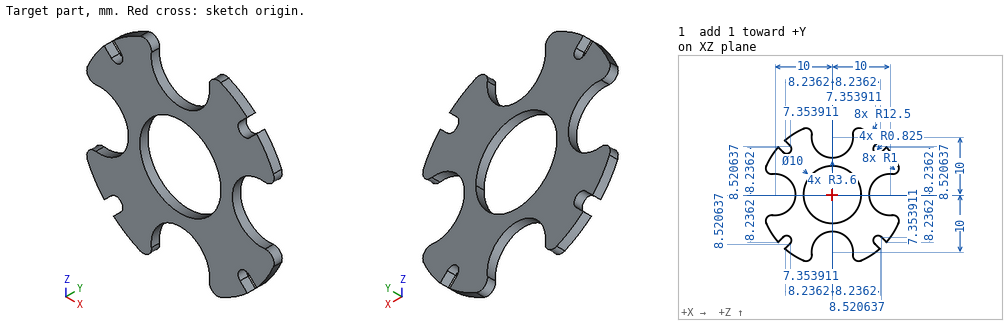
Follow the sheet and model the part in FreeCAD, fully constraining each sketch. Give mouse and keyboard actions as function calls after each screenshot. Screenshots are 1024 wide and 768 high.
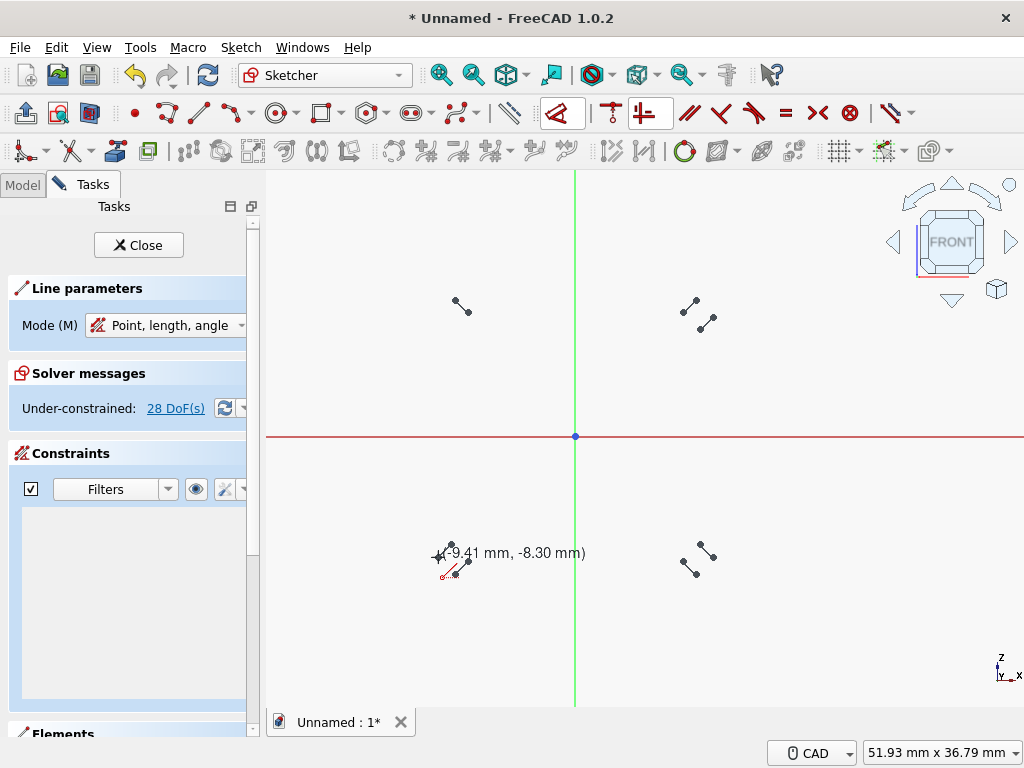
click(438, 317)
click(451, 329)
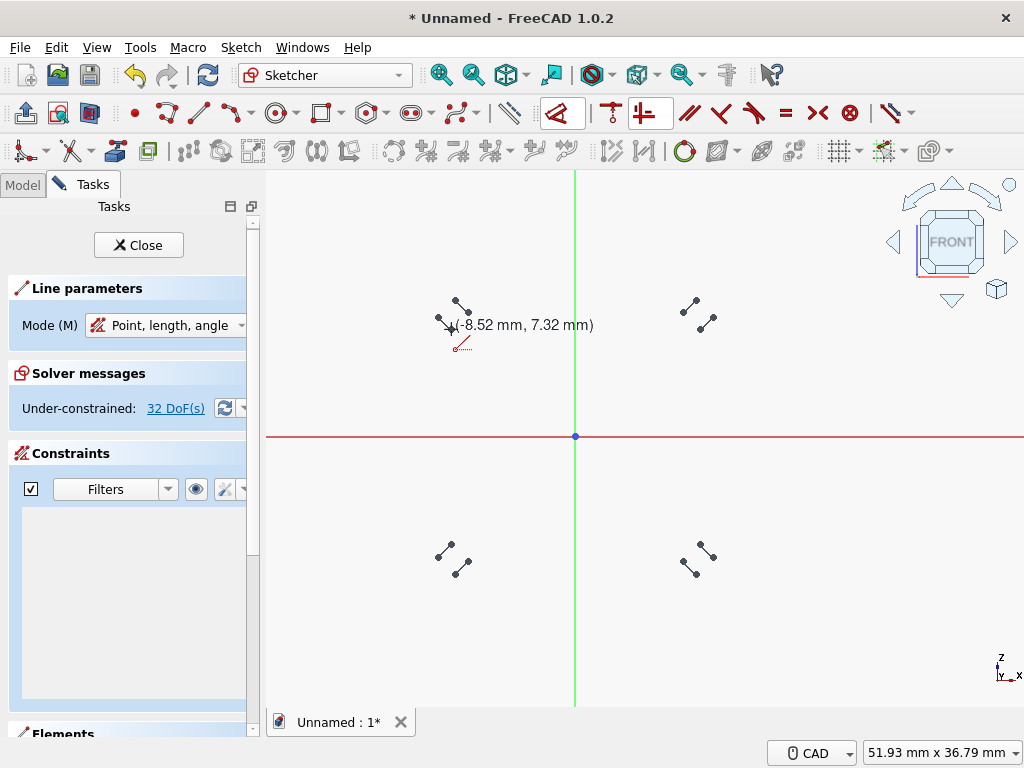
click(232, 114)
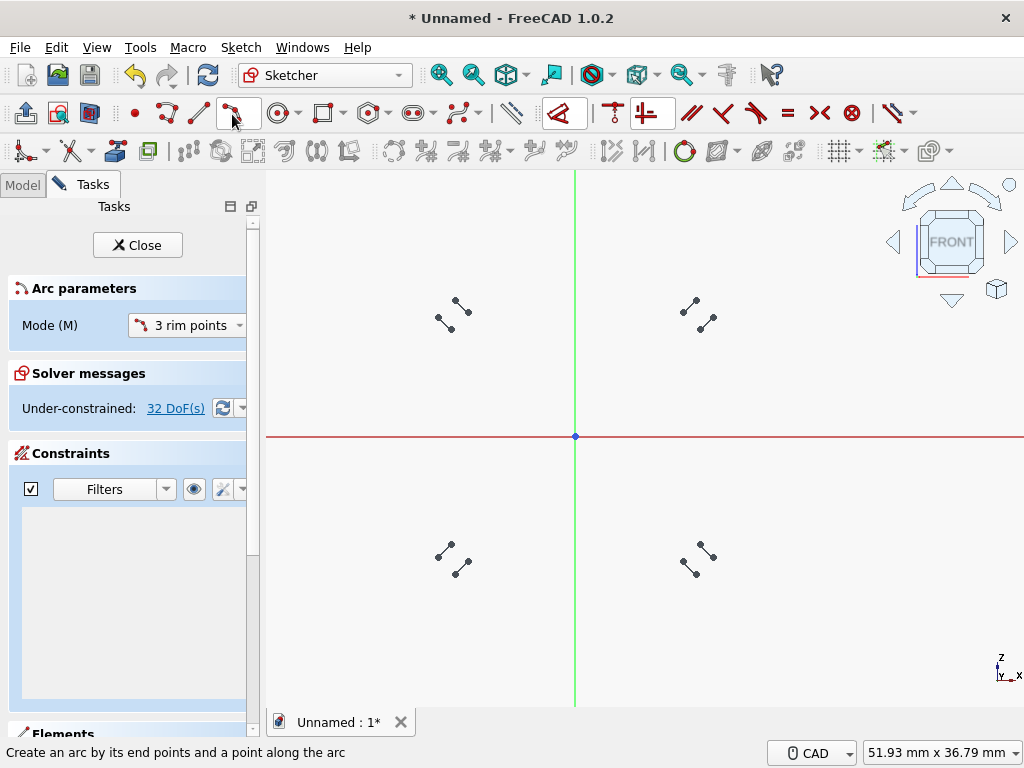
scroll(455, 300, up, 3)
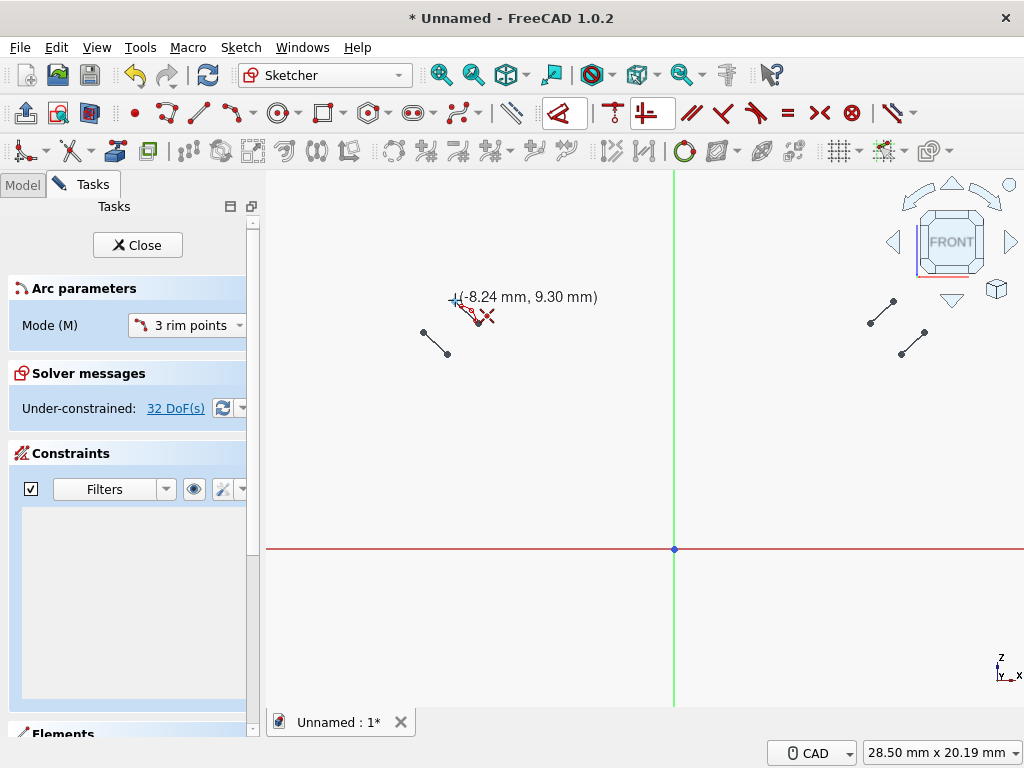
click(455, 302)
click(542, 244)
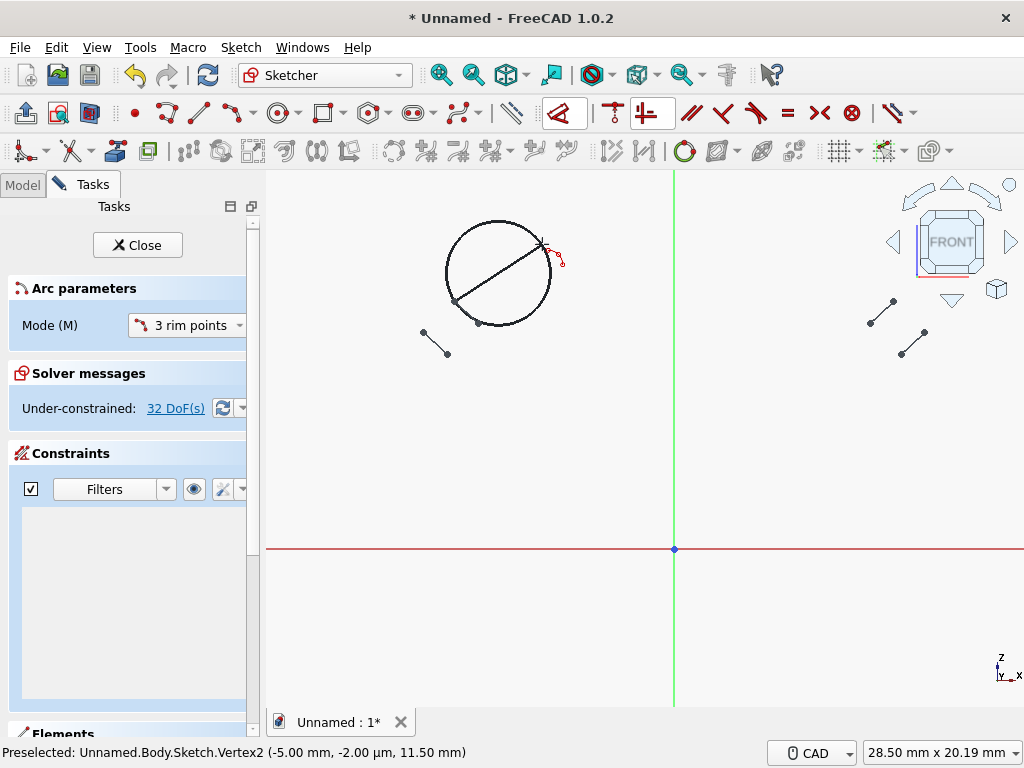
scroll(496, 268, up, 7)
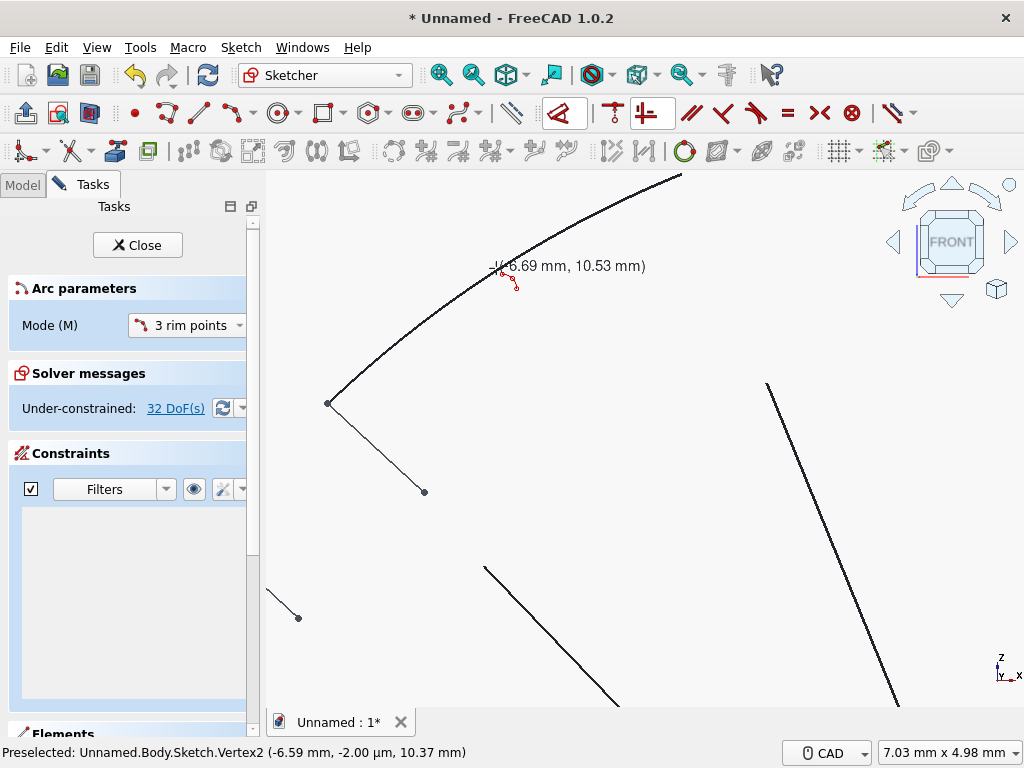
click(496, 268)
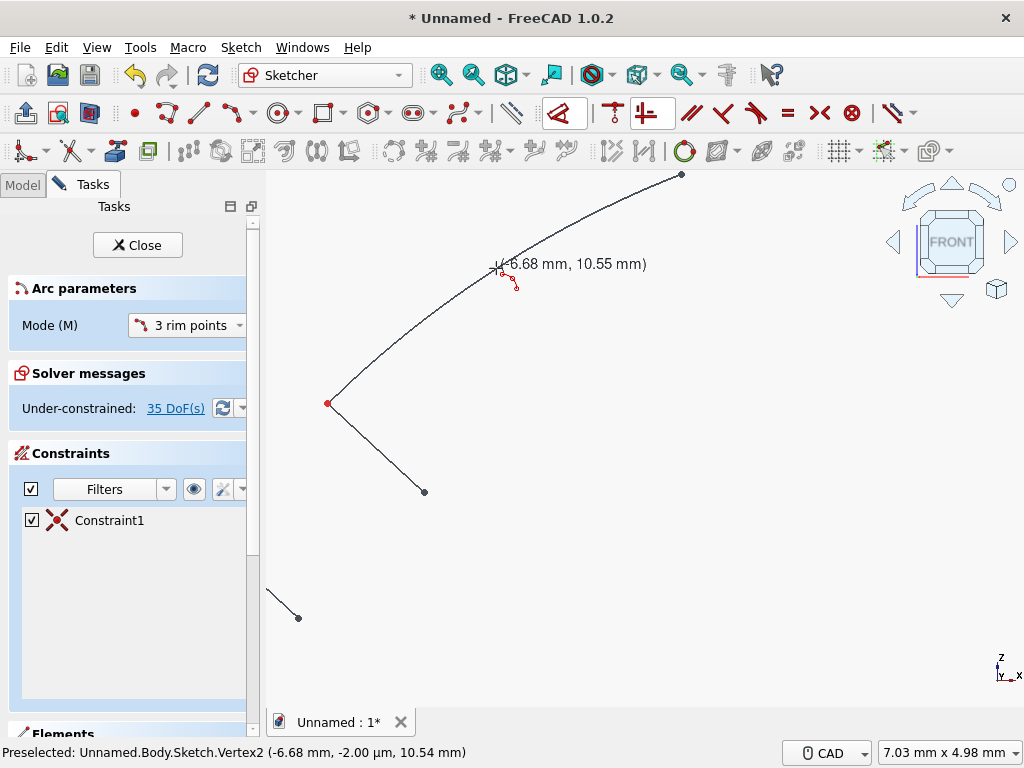
scroll(476, 287, down, 10)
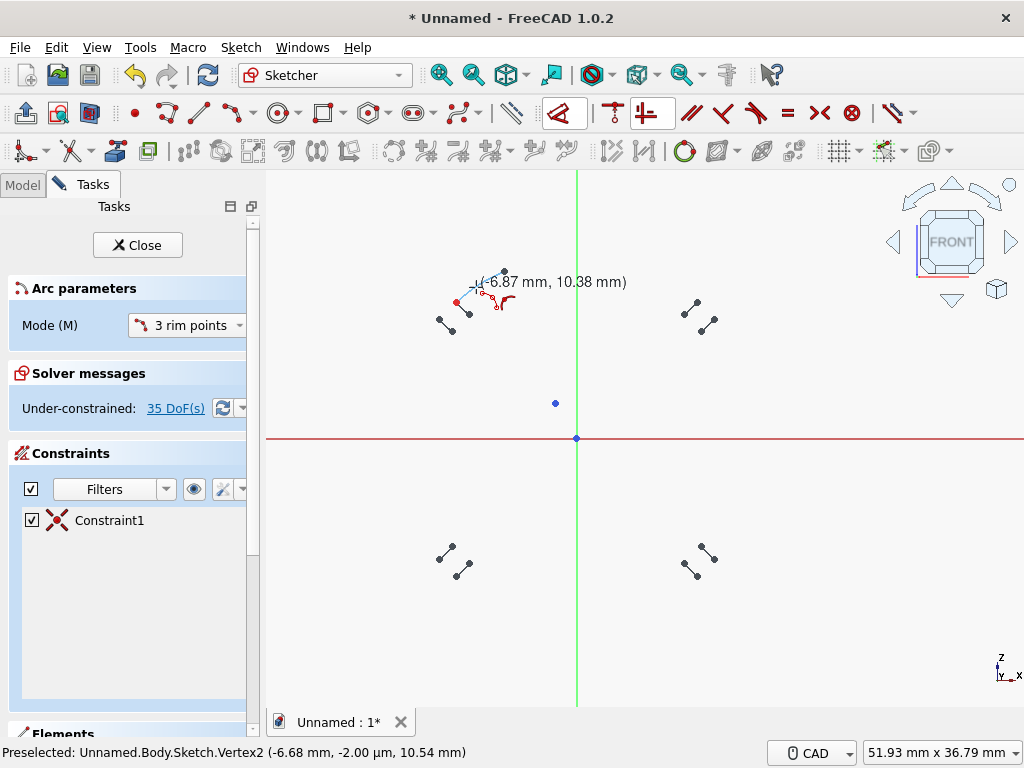
click(504, 272)
click(524, 286)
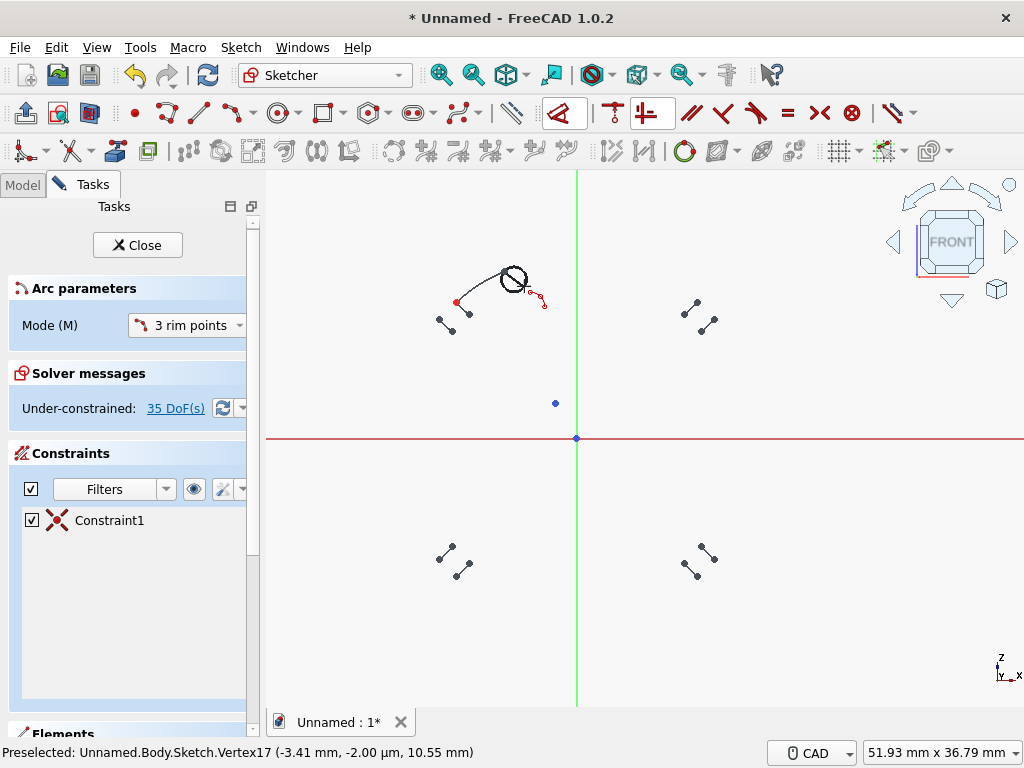
scroll(519, 273, up, 4)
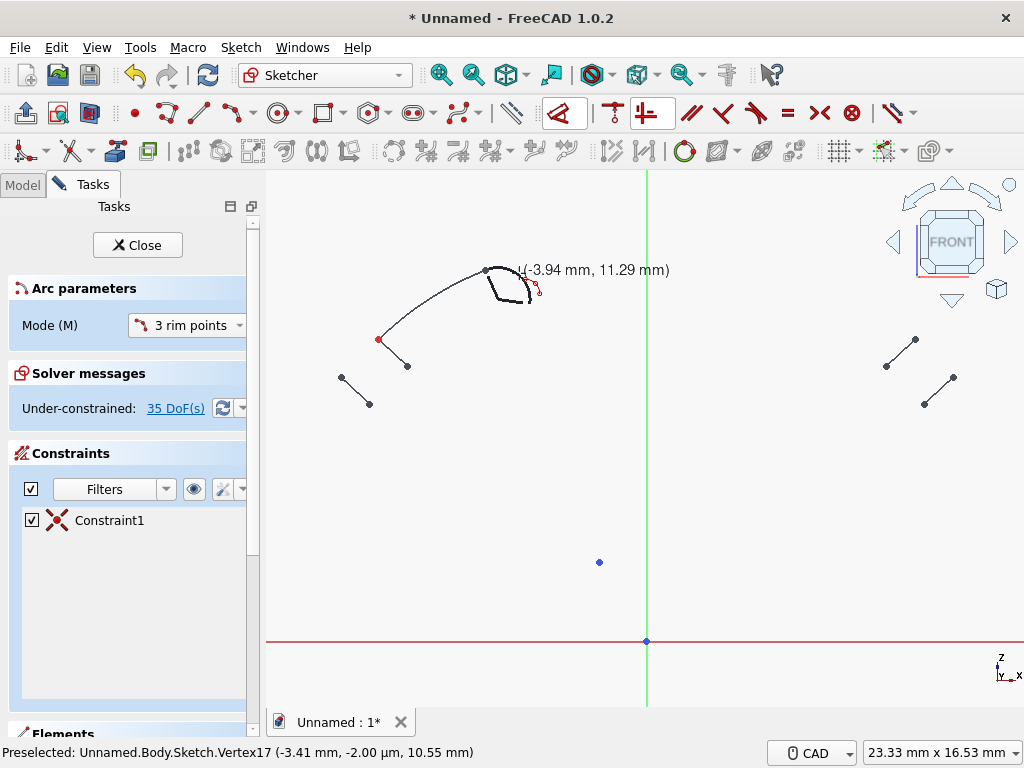
click(518, 273)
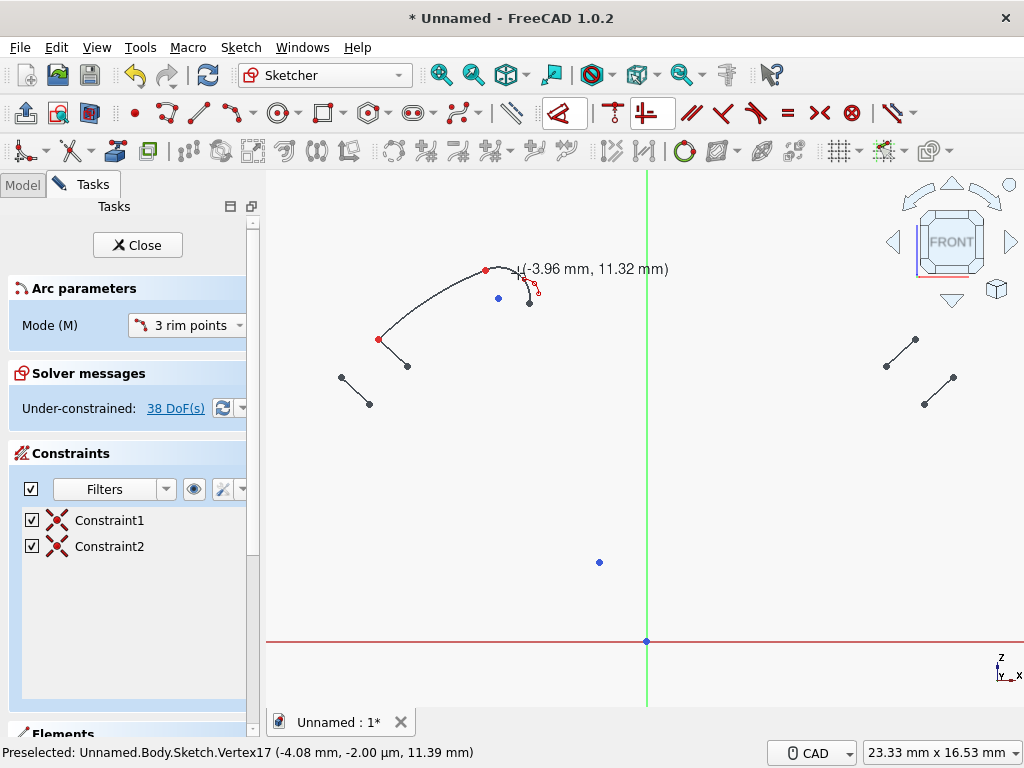
click(530, 304)
click(763, 303)
click(608, 427)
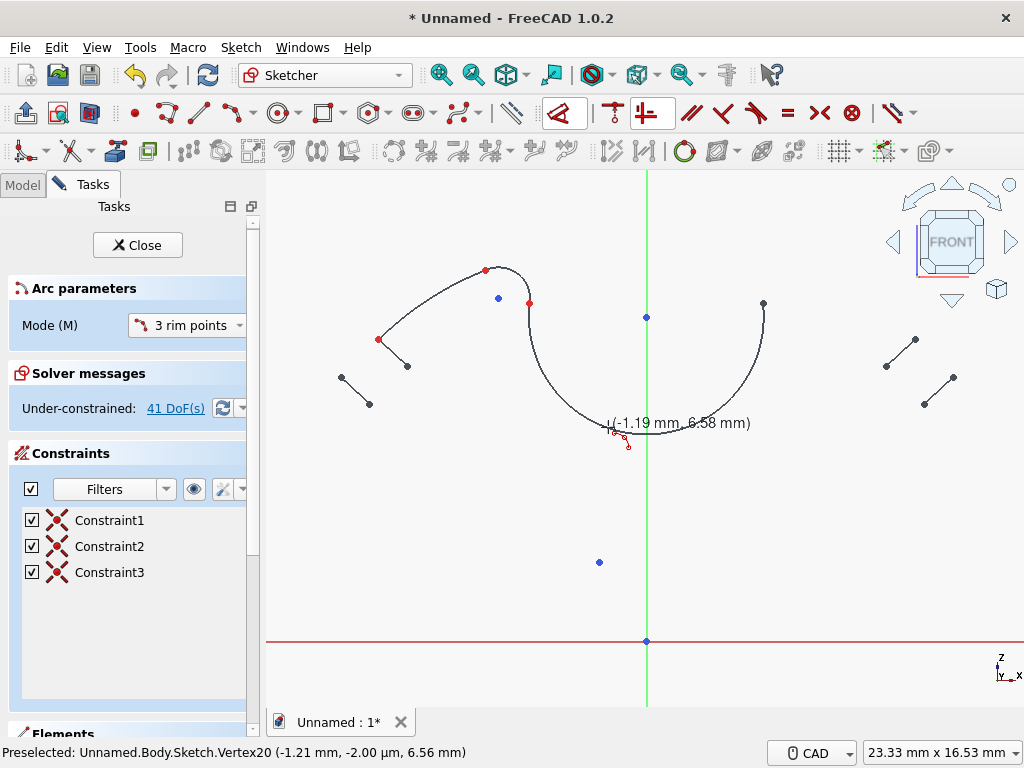
click(763, 304)
click(808, 269)
click(776, 273)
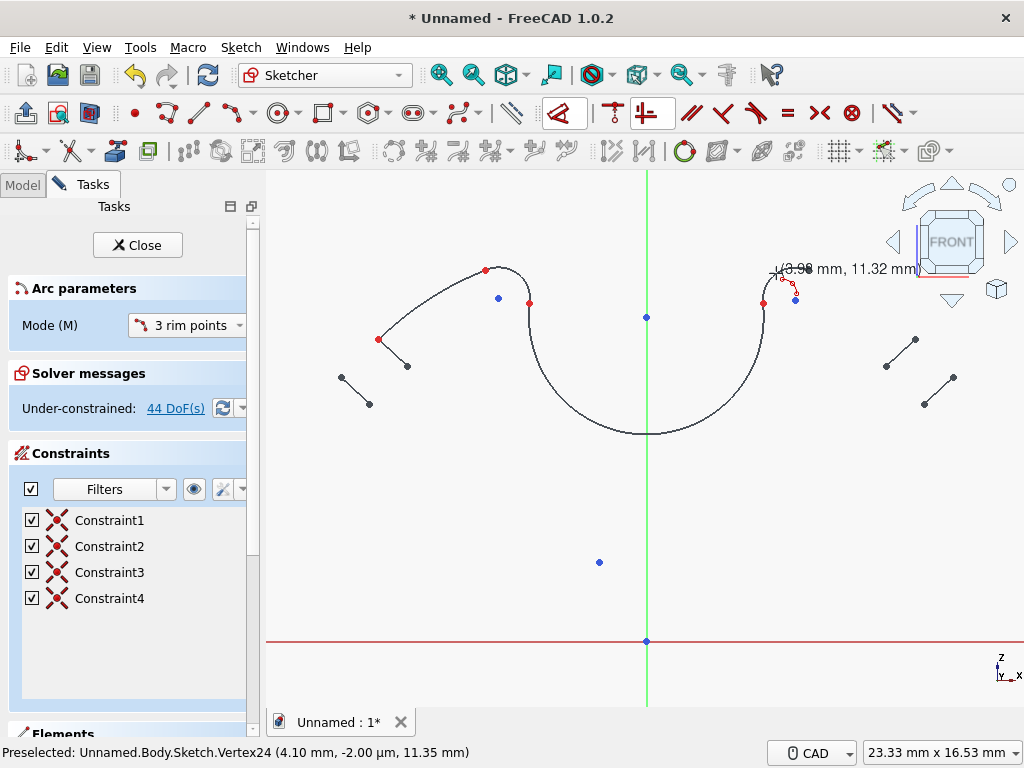
click(808, 270)